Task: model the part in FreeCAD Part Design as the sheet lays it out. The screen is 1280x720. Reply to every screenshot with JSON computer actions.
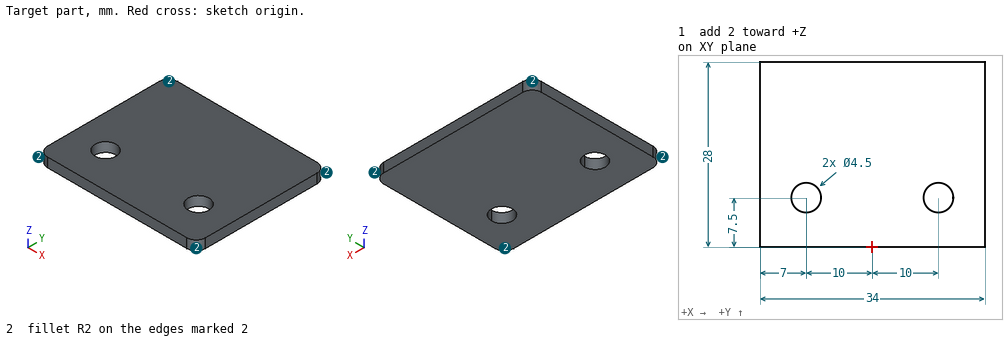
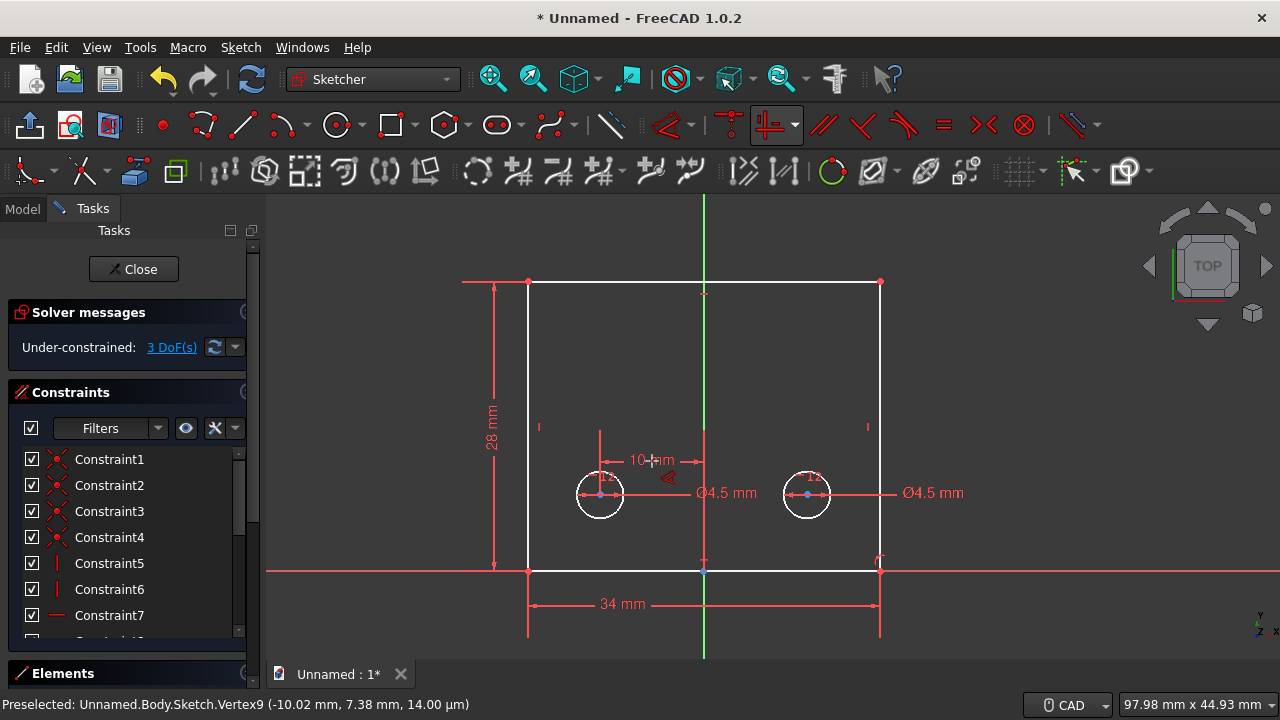
{"action": "left_click", "coordinate": [807, 495]}
{"action": "left_click", "coordinate": [755, 605]}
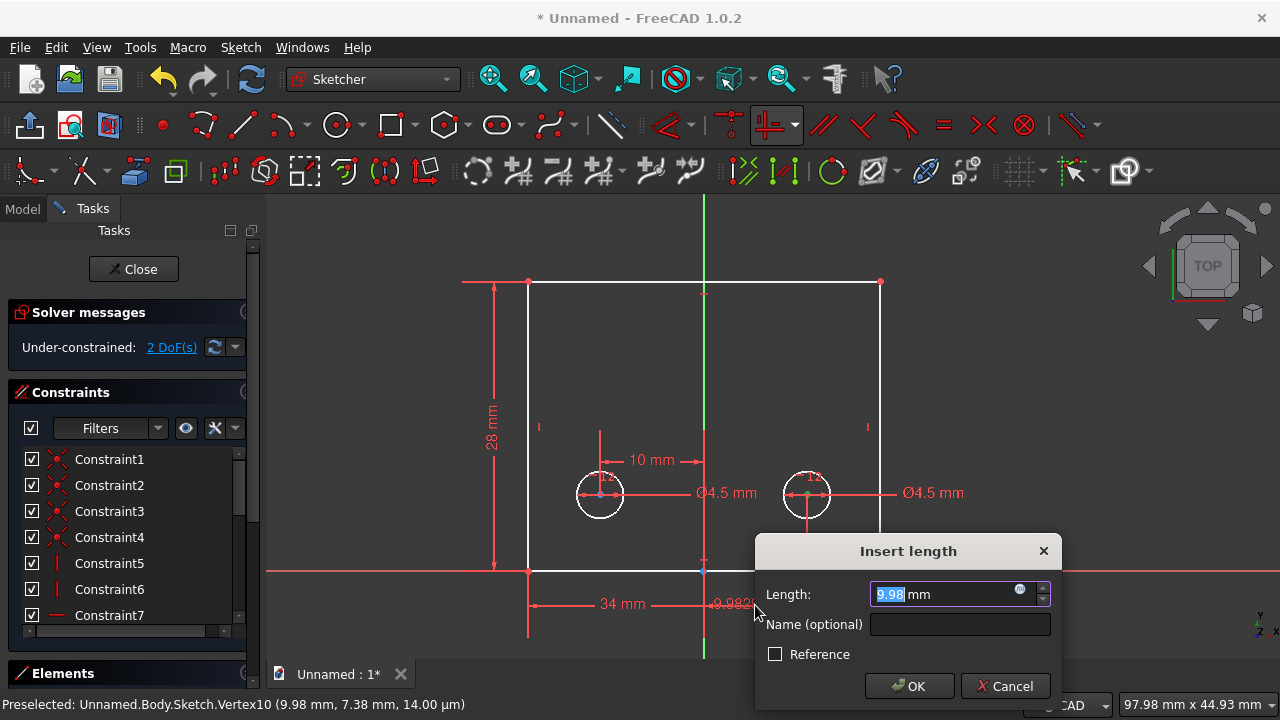
{"action": "type", "text": "10"}
{"action": "key", "text": "Return"}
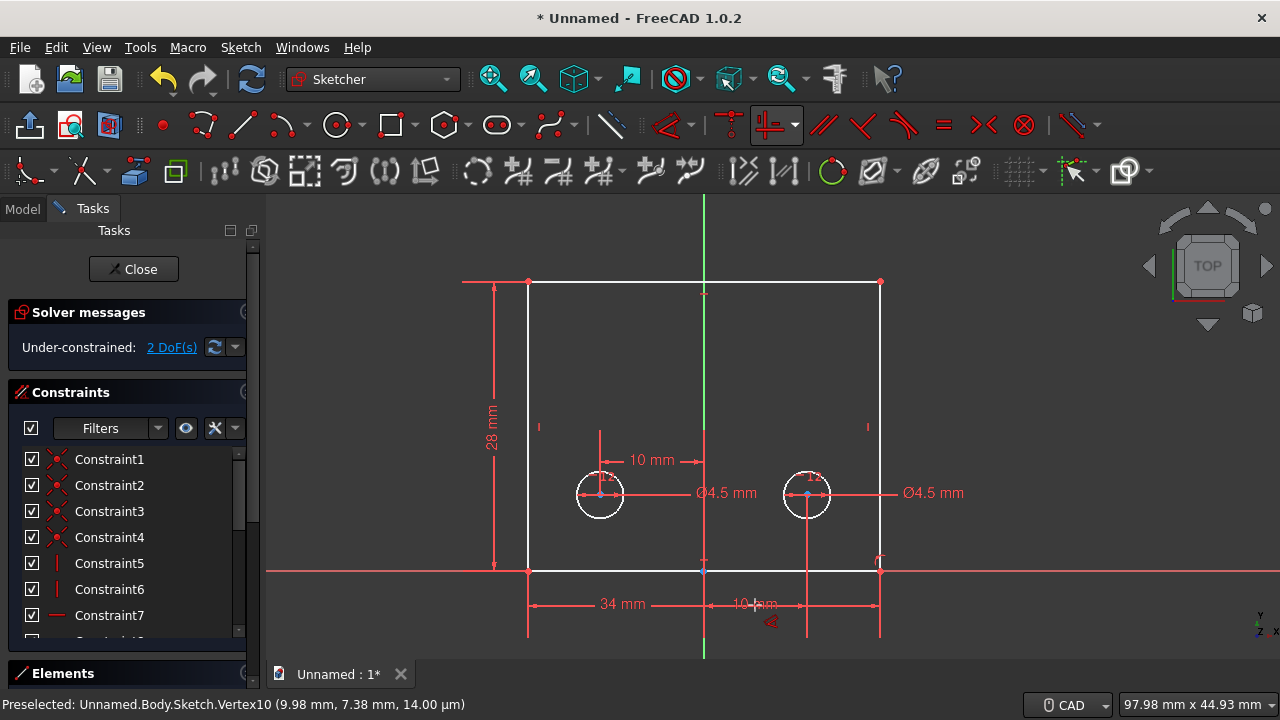
{"action": "left_click", "coordinate": [528, 571]}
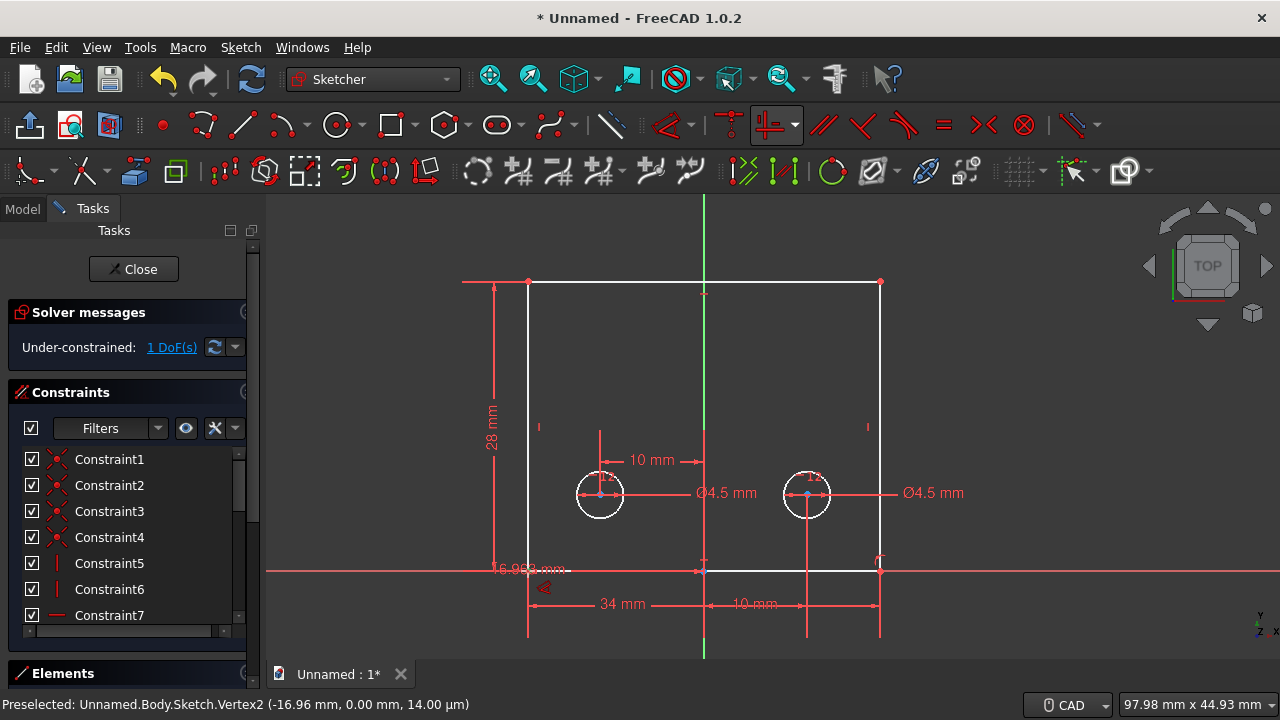
{"action": "left_click", "coordinate": [600, 495]}
{"action": "left_click", "coordinate": [548, 605]}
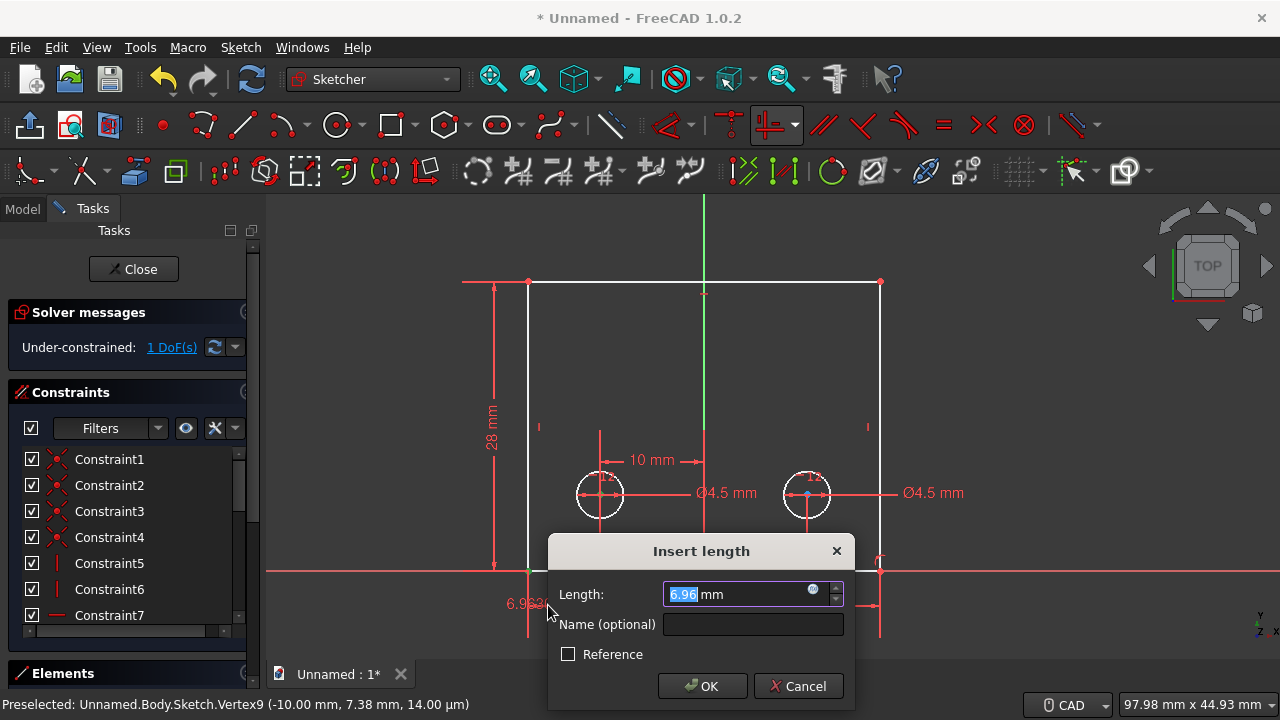
{"action": "type", "text": "7"}
{"action": "key", "text": "Return"}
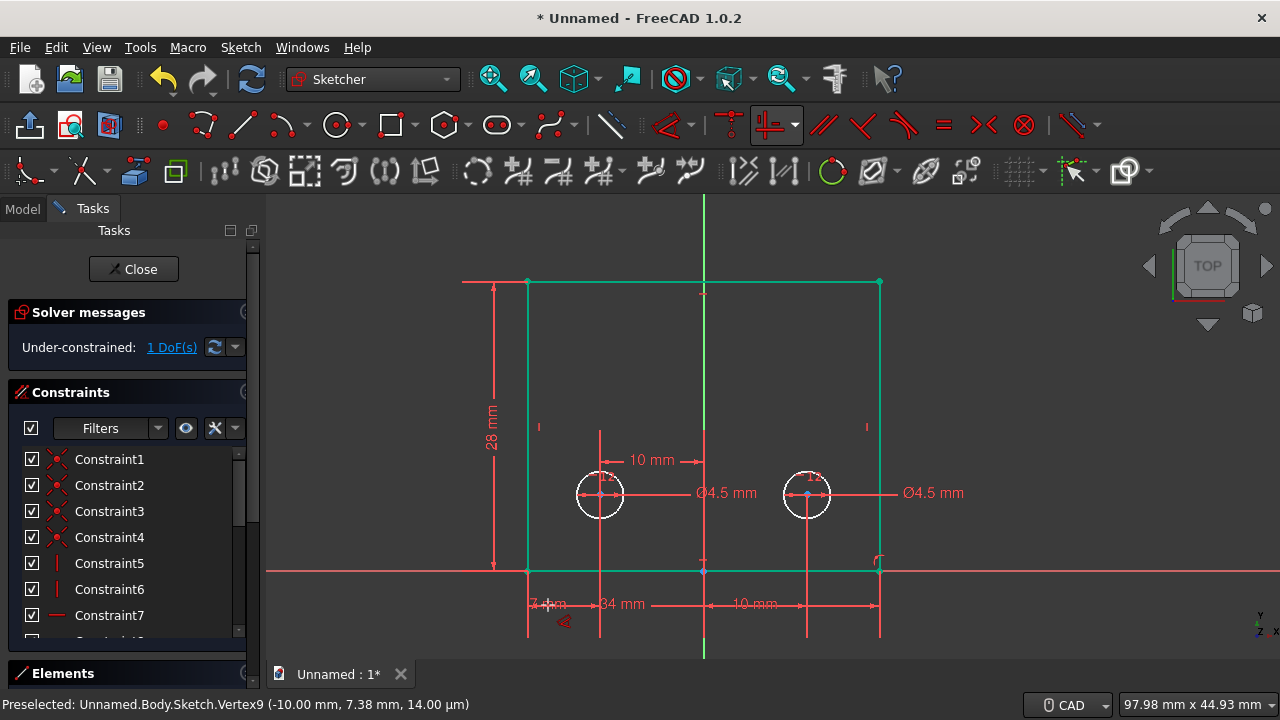
{"action": "left_click", "coordinate": [600, 495]}
{"action": "left_click", "coordinate": [566, 533]}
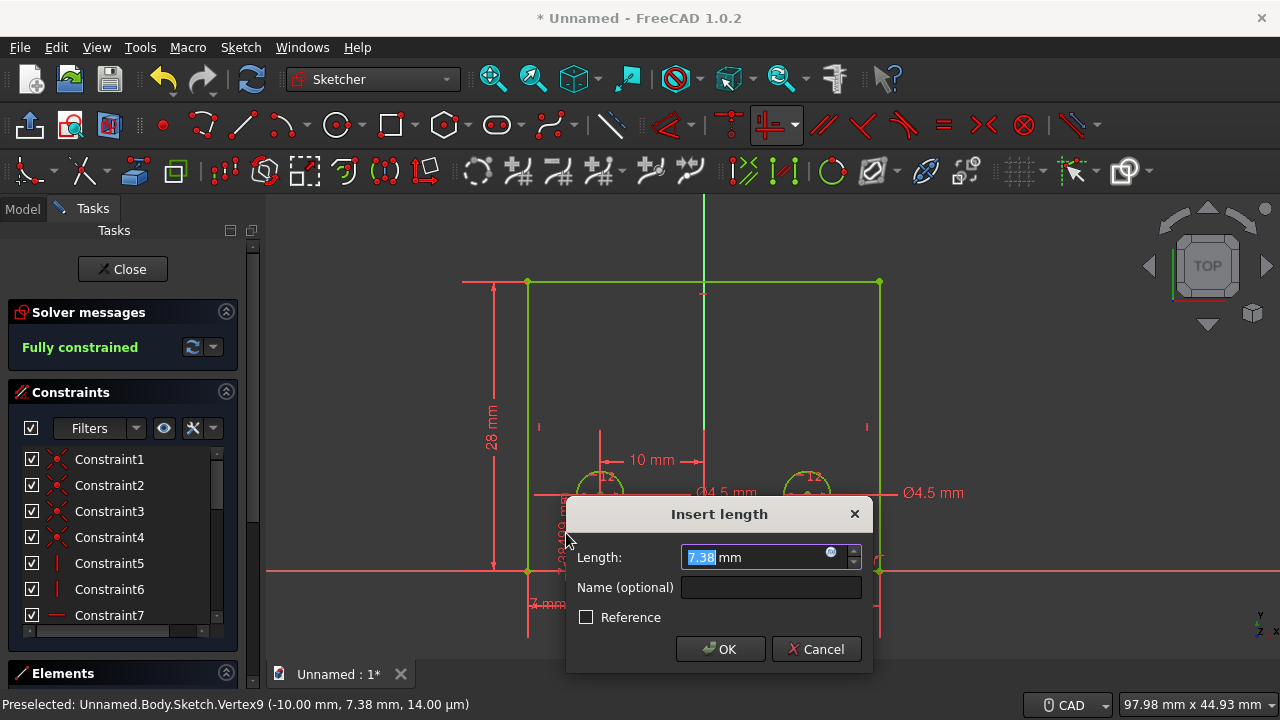
{"action": "type", "text": "7.5"}
{"action": "key", "text": "Return"}
{"action": "key", "text": "Escape"}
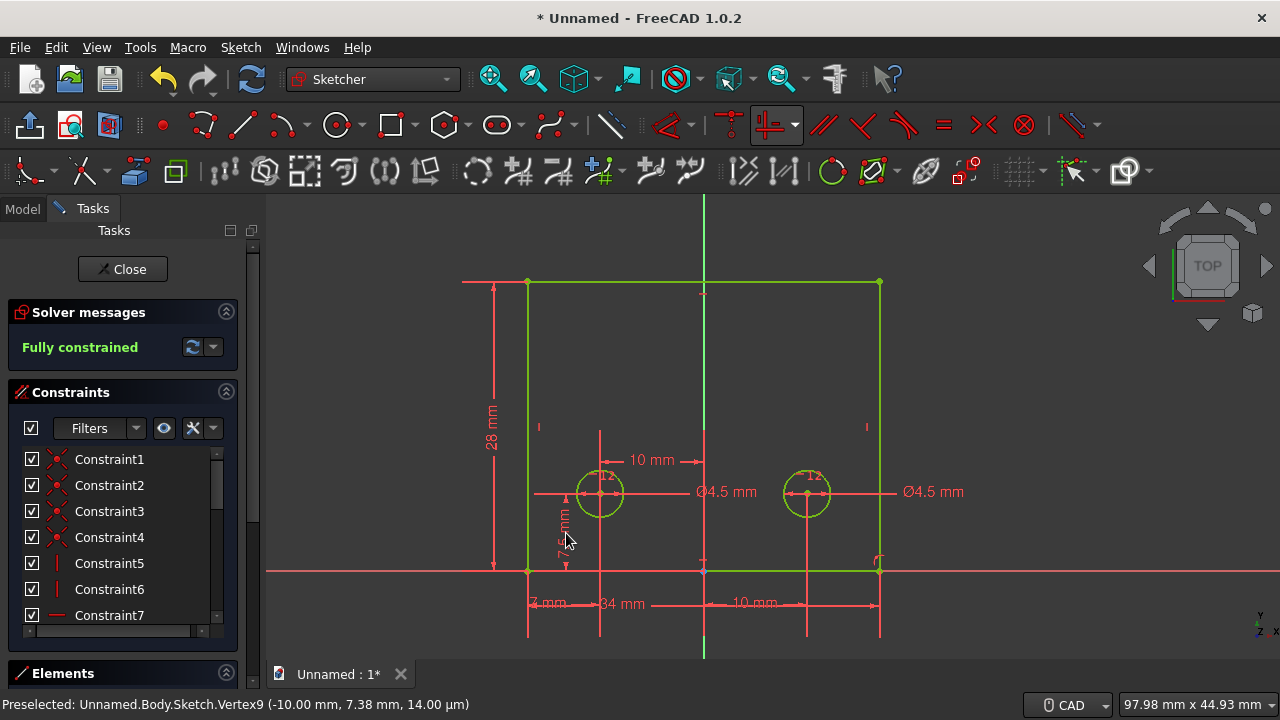
{"action": "left_click", "coordinate": [123, 269]}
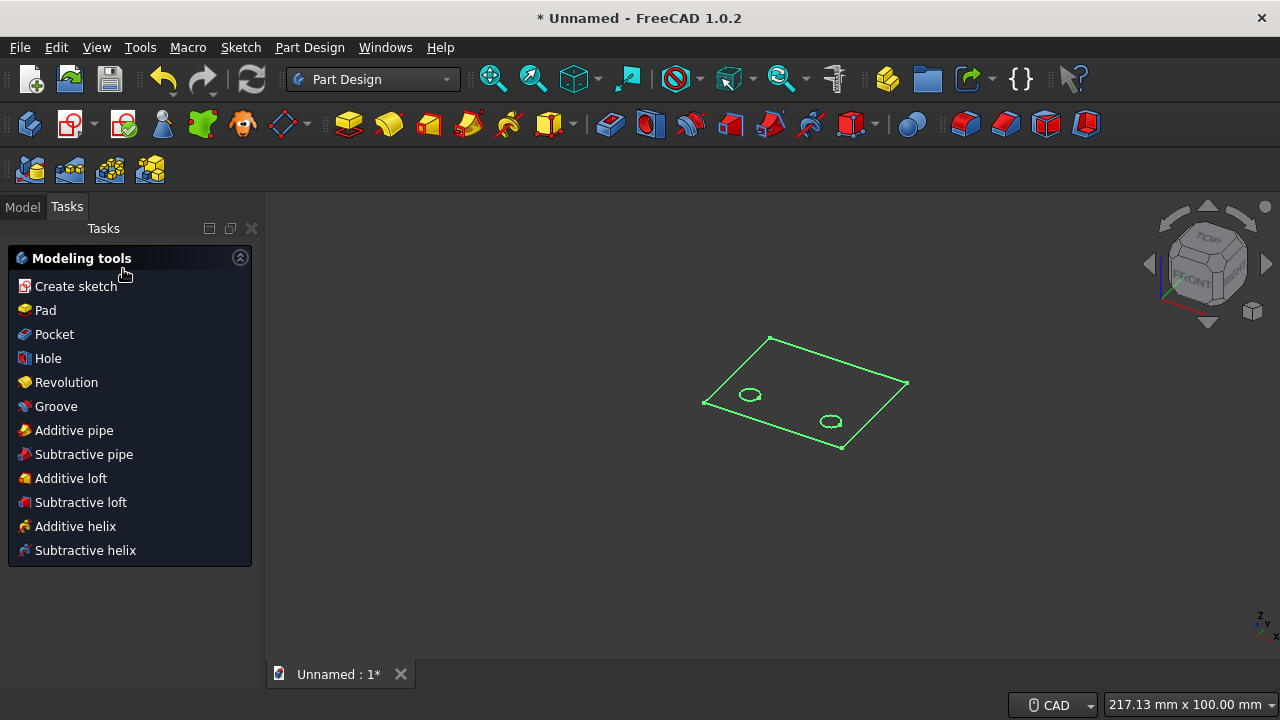
{"action": "left_click", "coordinate": [350, 124]}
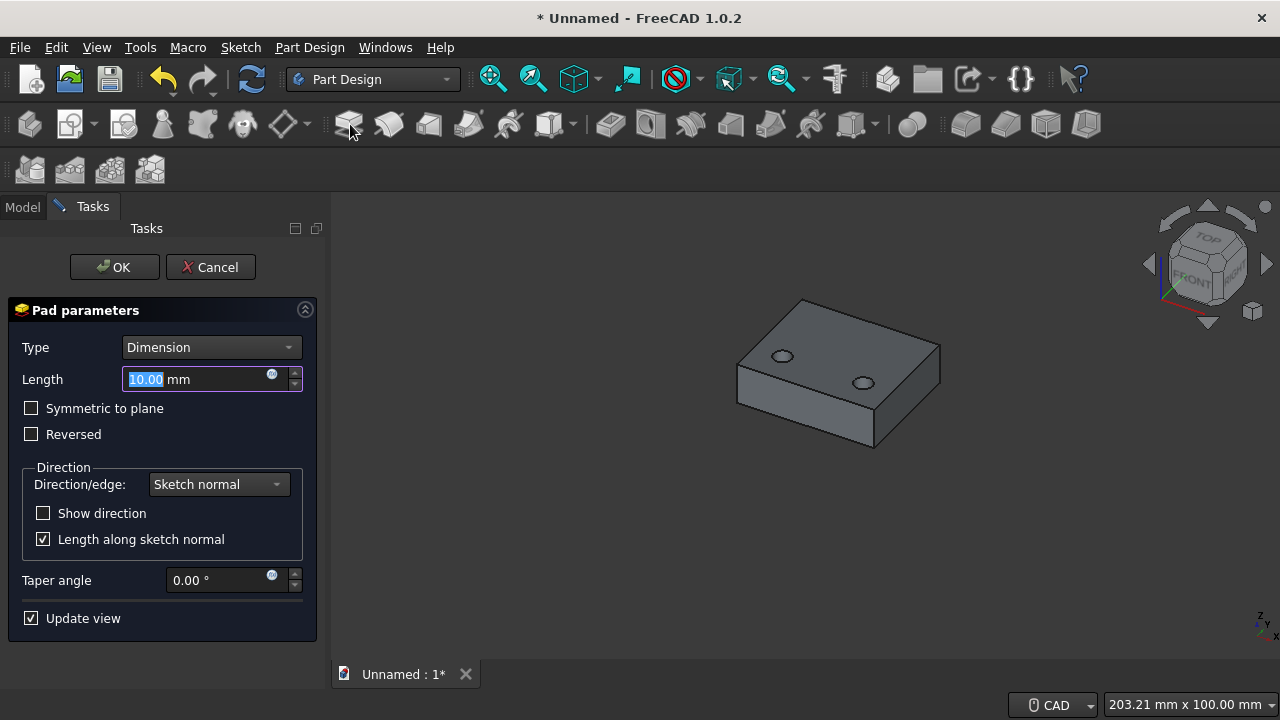
{"action": "type", "text": "2"}
{"action": "key", "text": "Tab"}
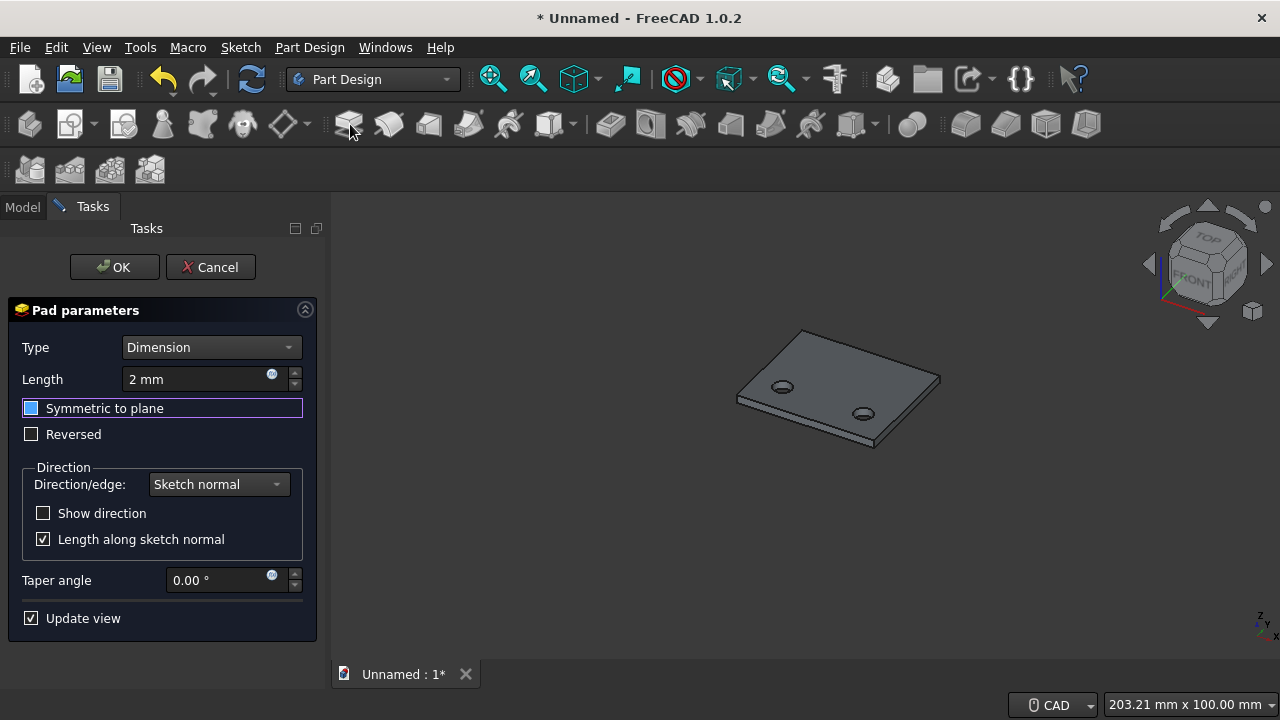
{"action": "left_click", "coordinate": [115, 267]}